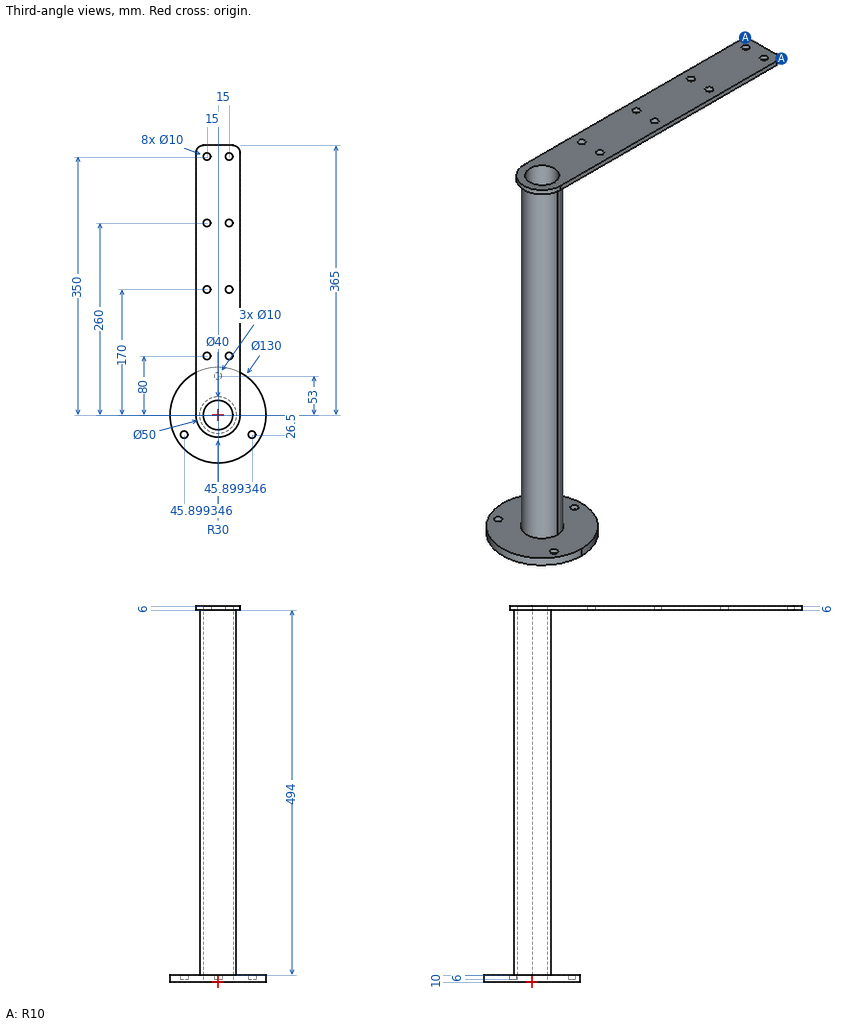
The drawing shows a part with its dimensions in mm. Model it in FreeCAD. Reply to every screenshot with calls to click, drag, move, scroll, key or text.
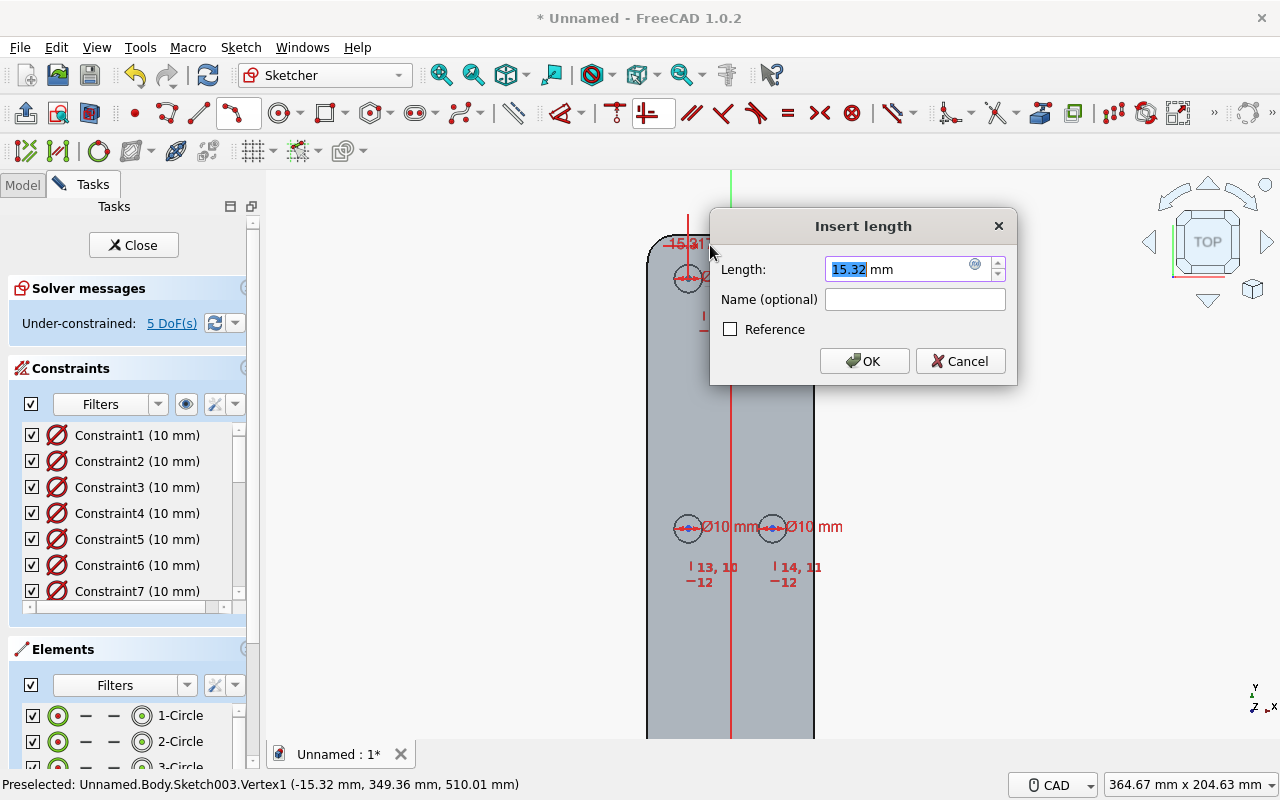
text(15)
key(Return)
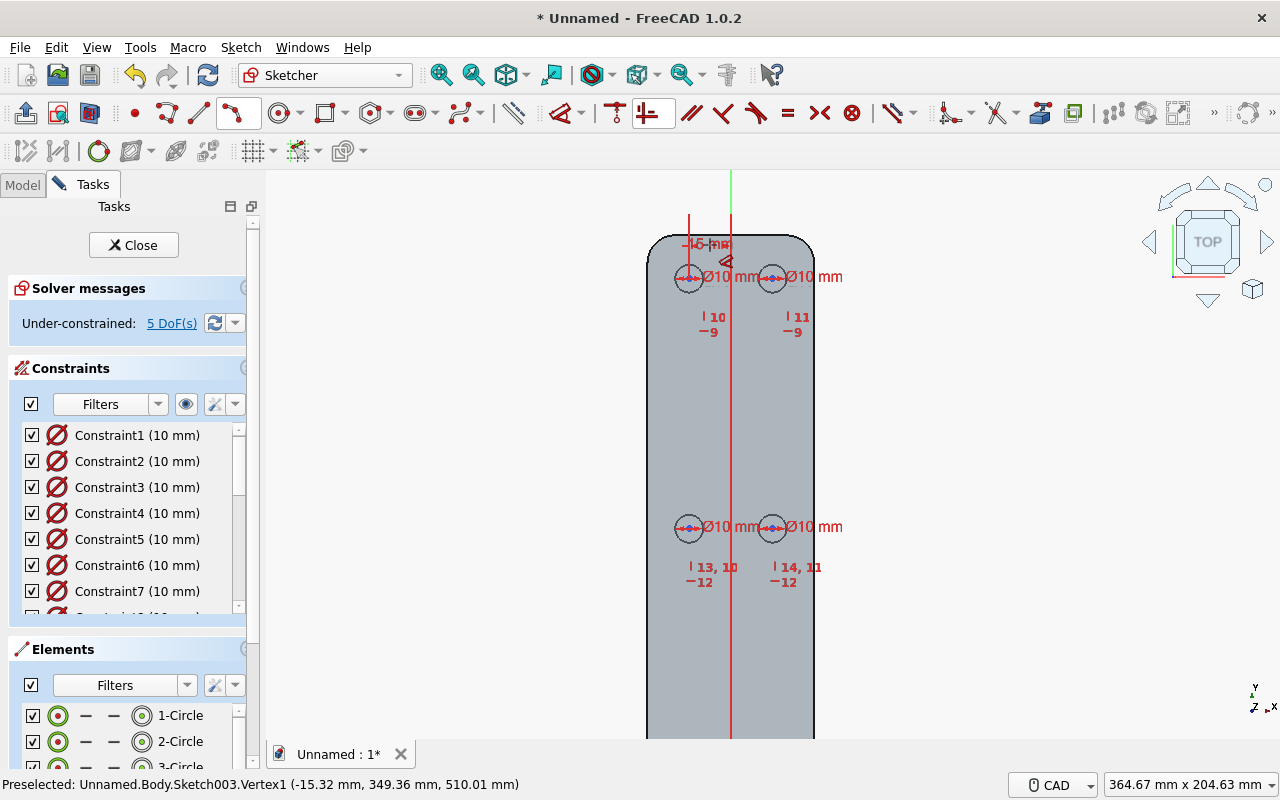
click(773, 279)
click(752, 221)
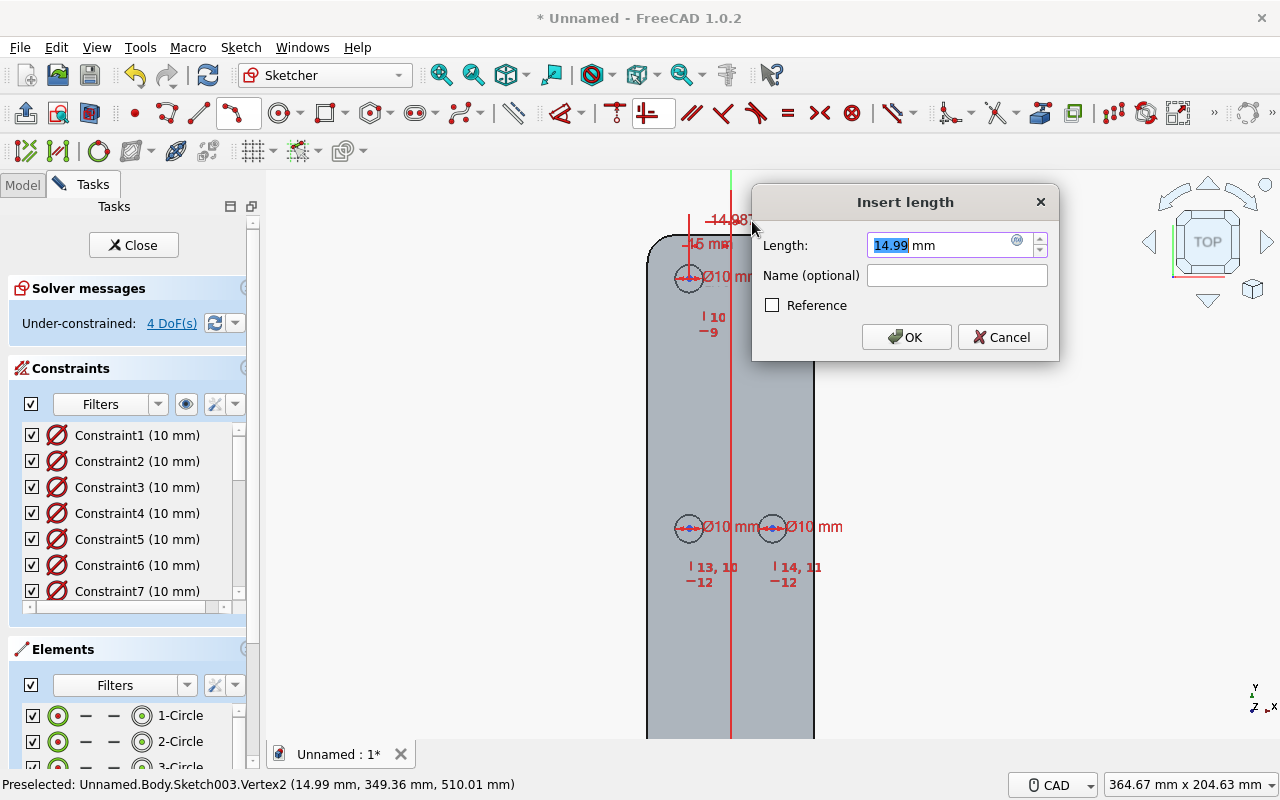
text(15)
key(Return)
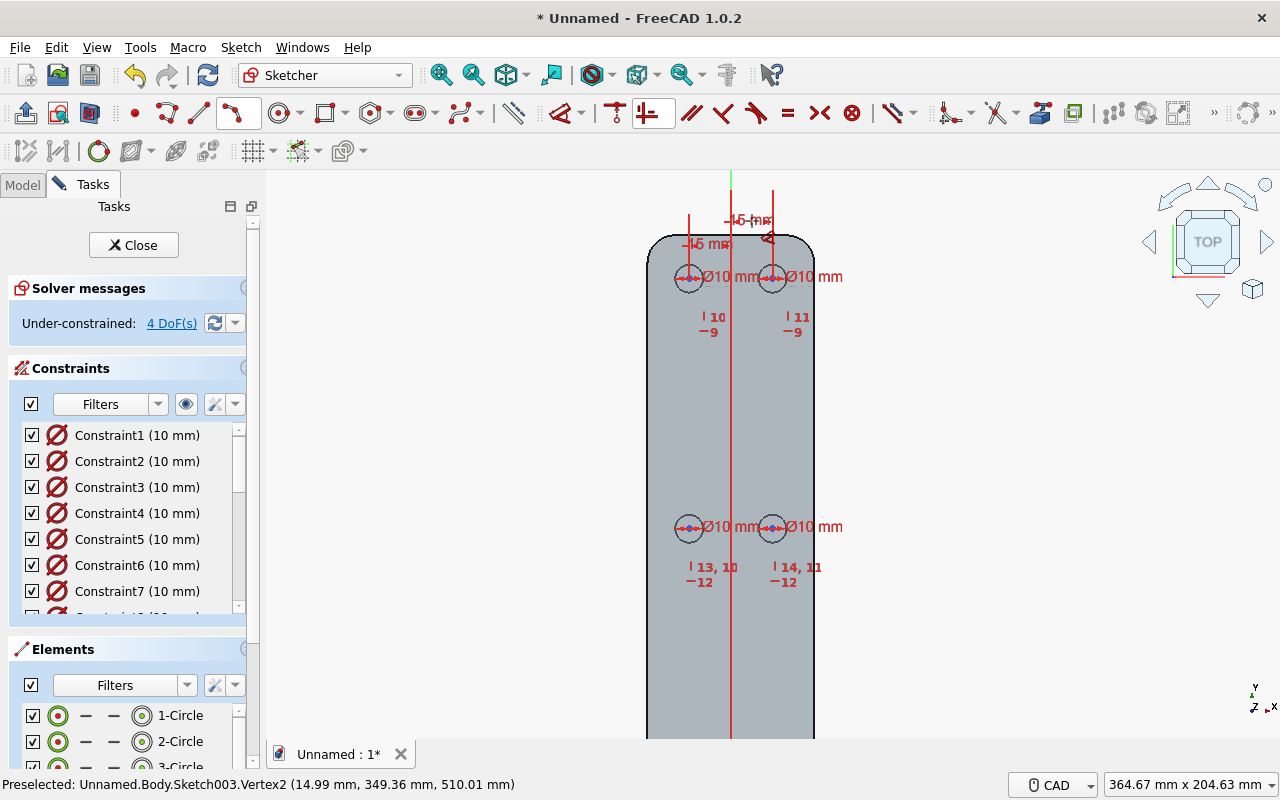
scroll(689, 279, down, 5)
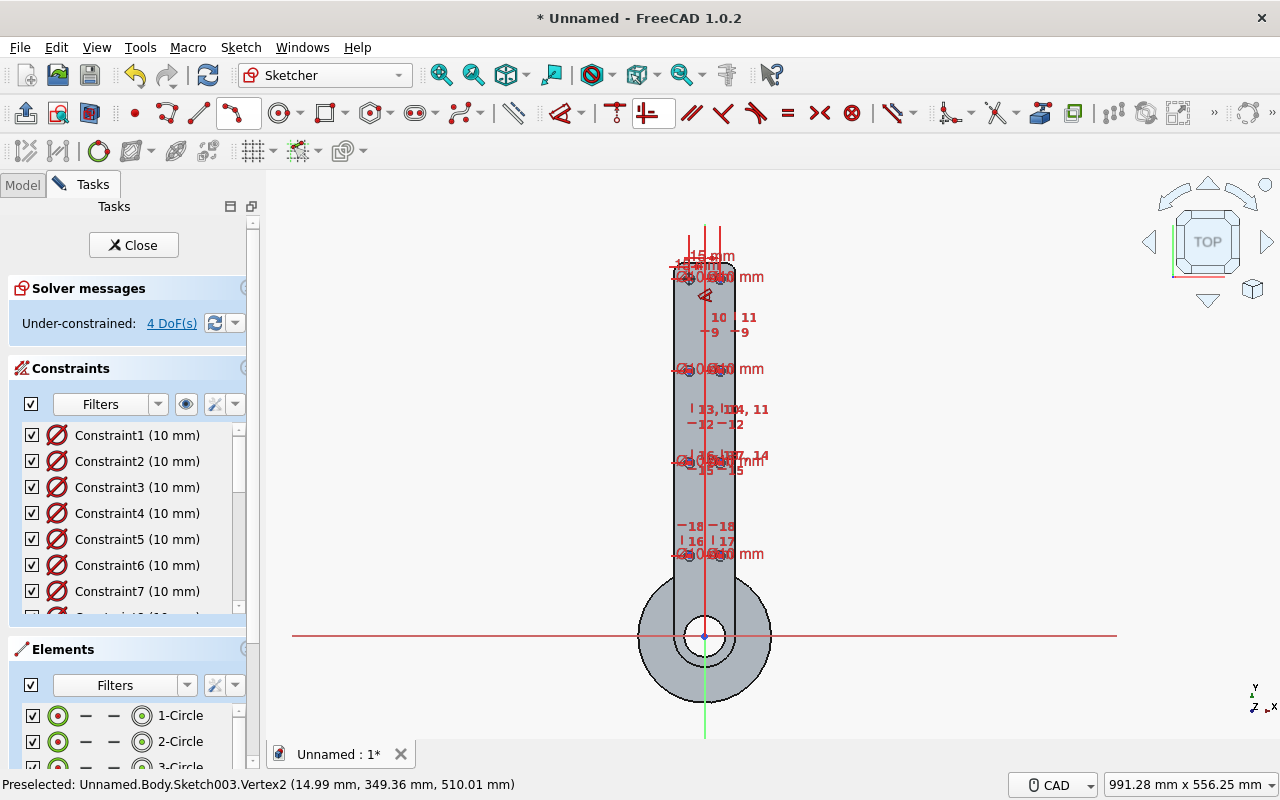
click(689, 556)
click(655, 596)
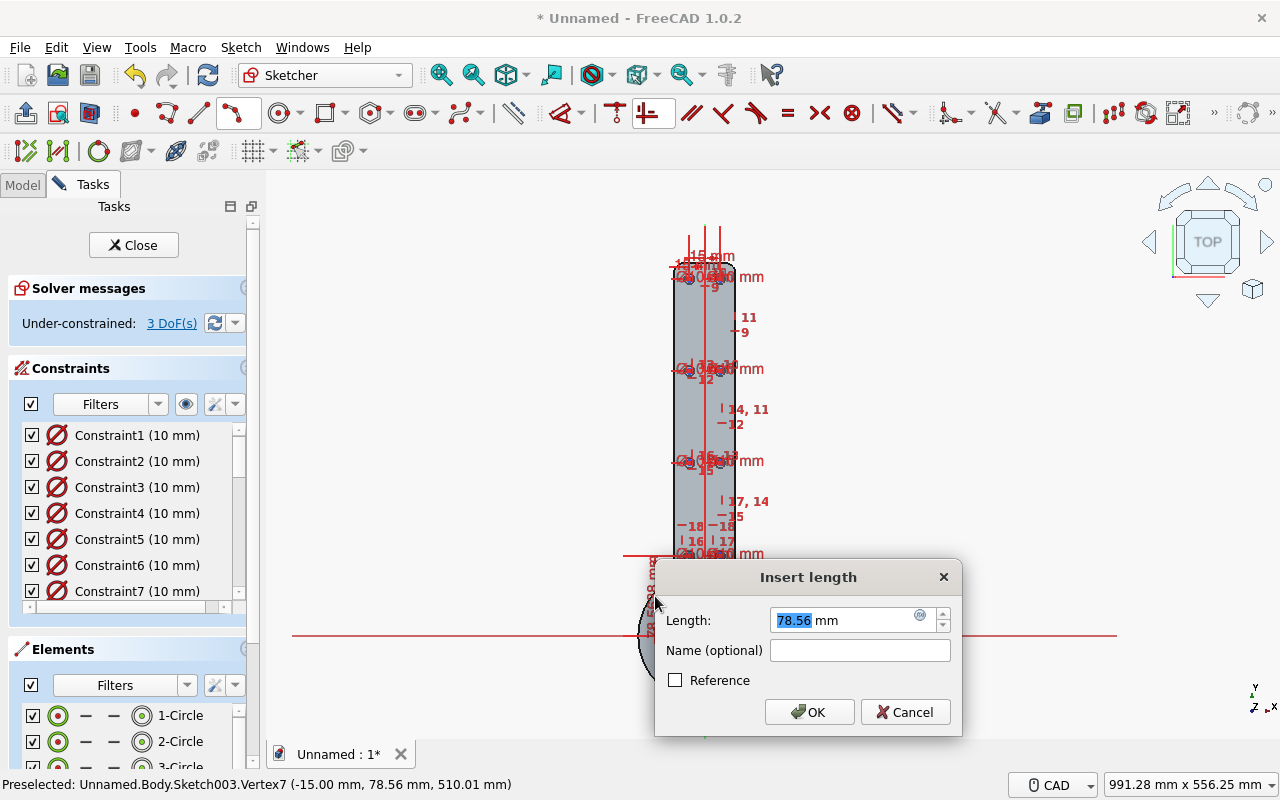
text(80)
key(Return)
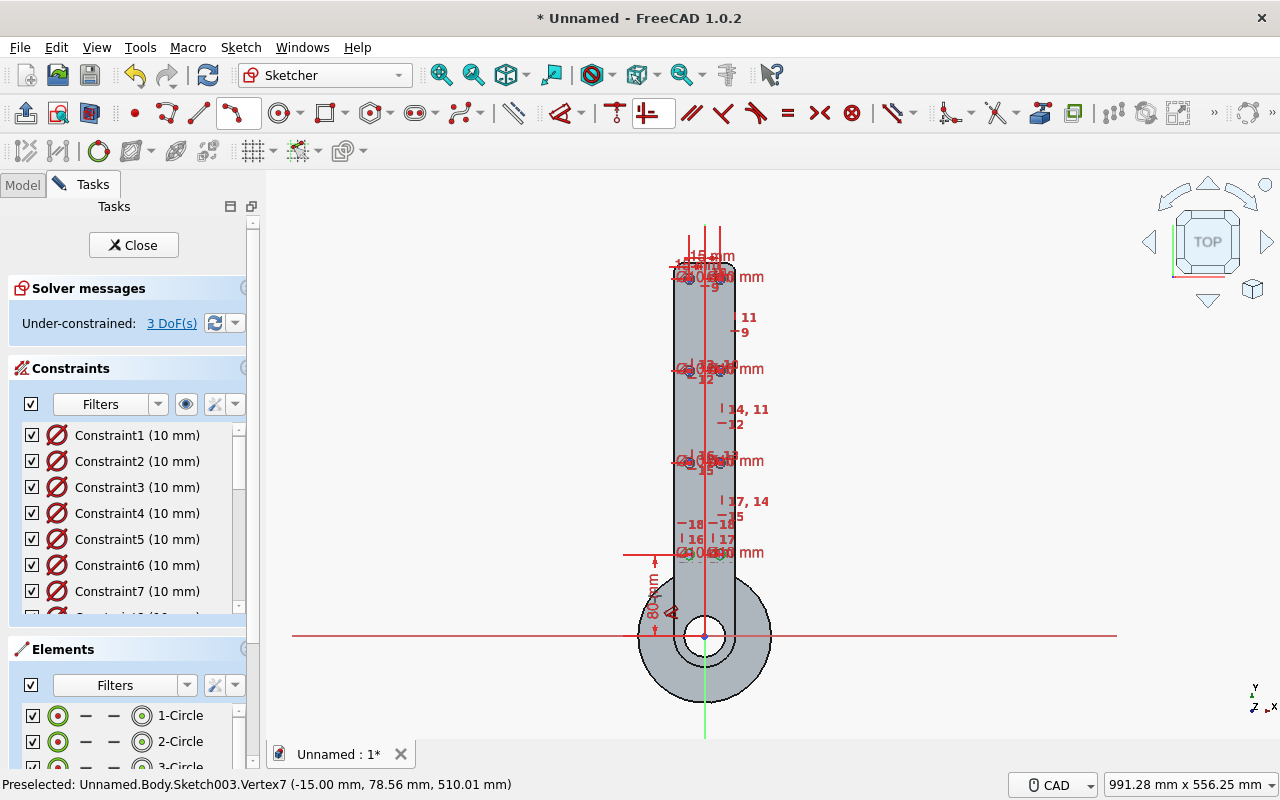
click(689, 279)
click(655, 458)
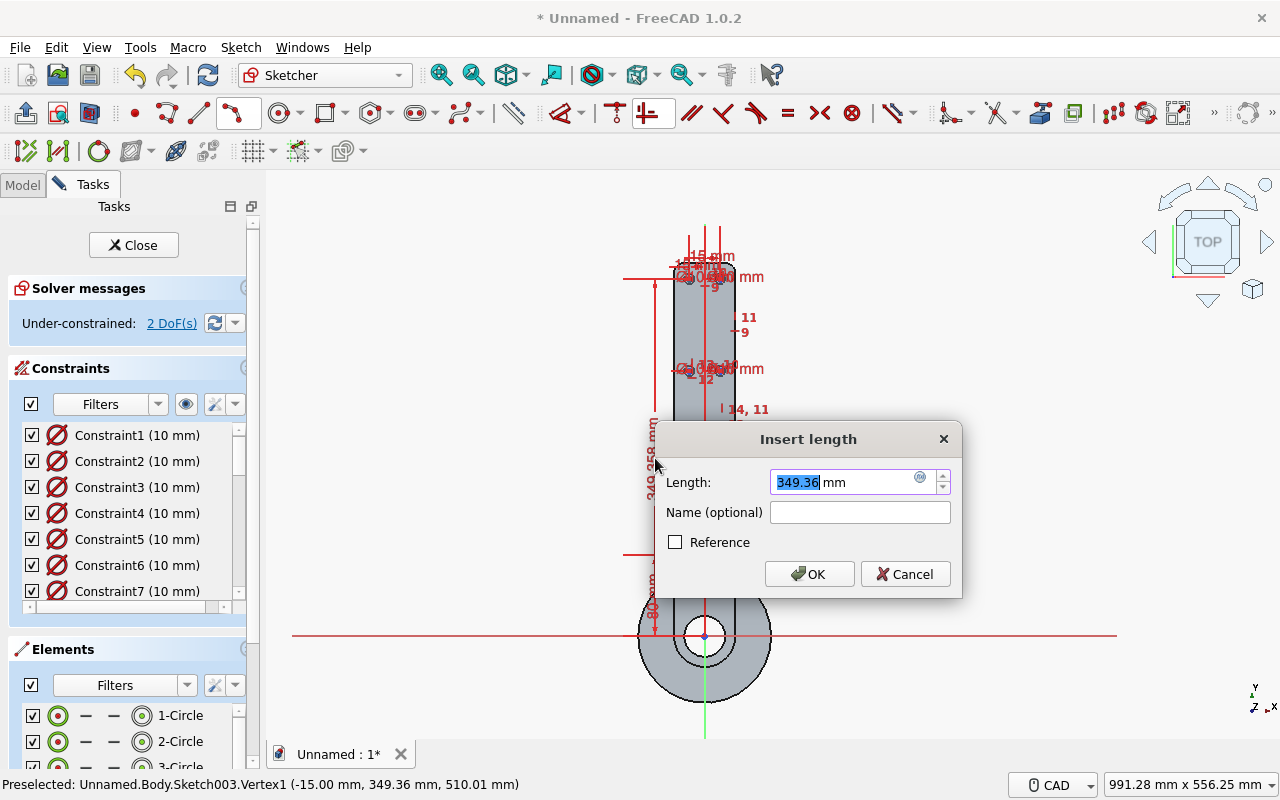
text(350)
key(Return)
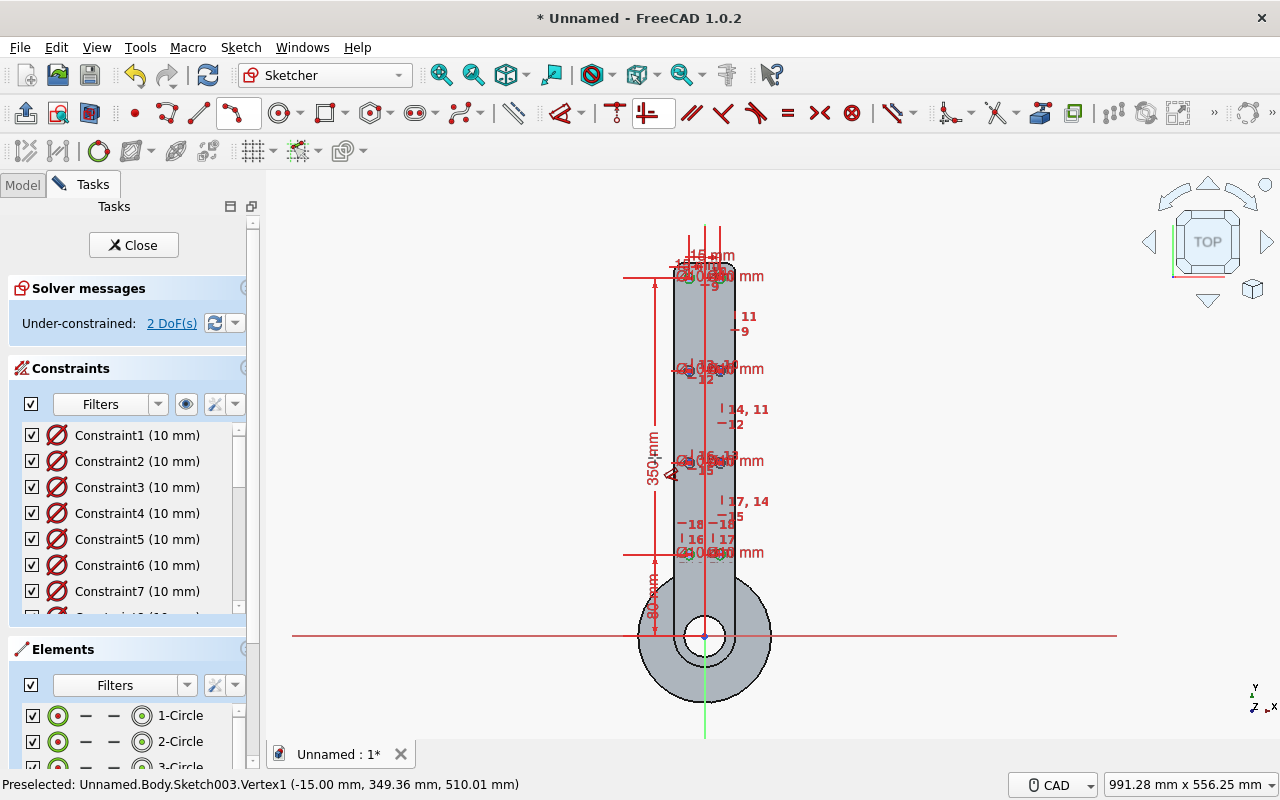
click(689, 371)
click(655, 504)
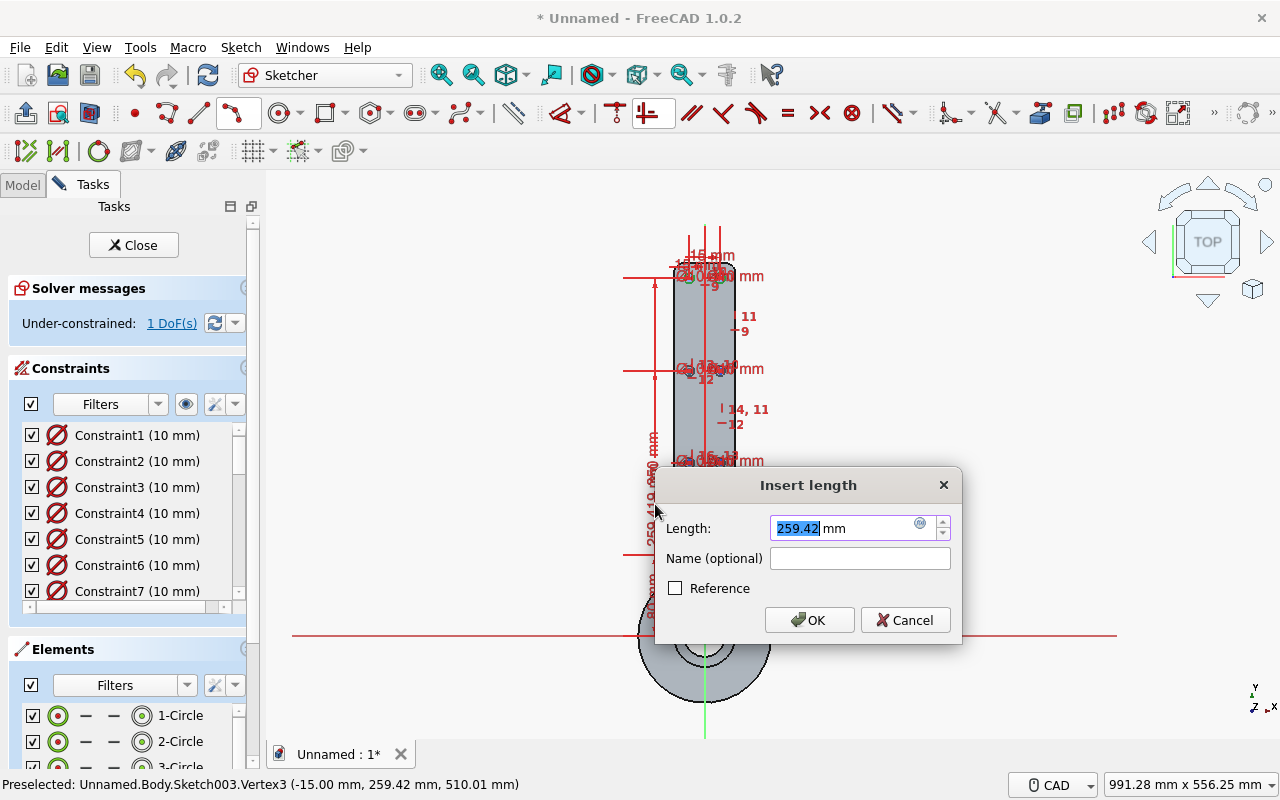
text(260)
key(Return)